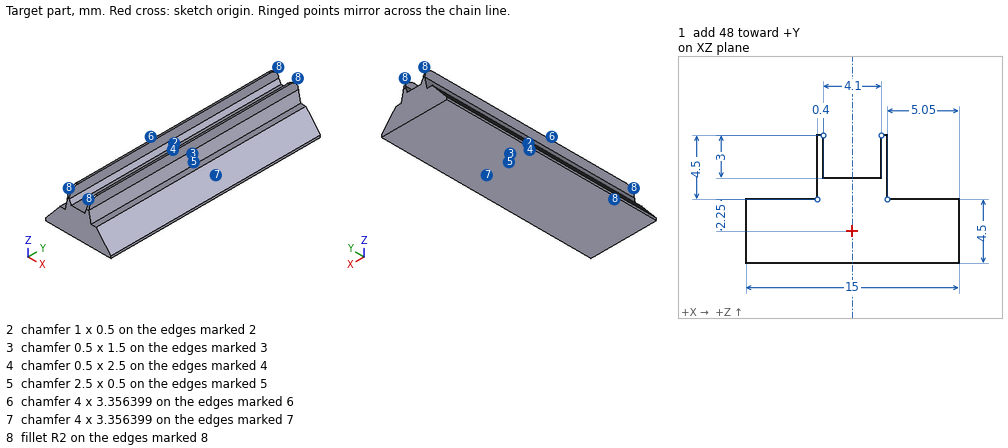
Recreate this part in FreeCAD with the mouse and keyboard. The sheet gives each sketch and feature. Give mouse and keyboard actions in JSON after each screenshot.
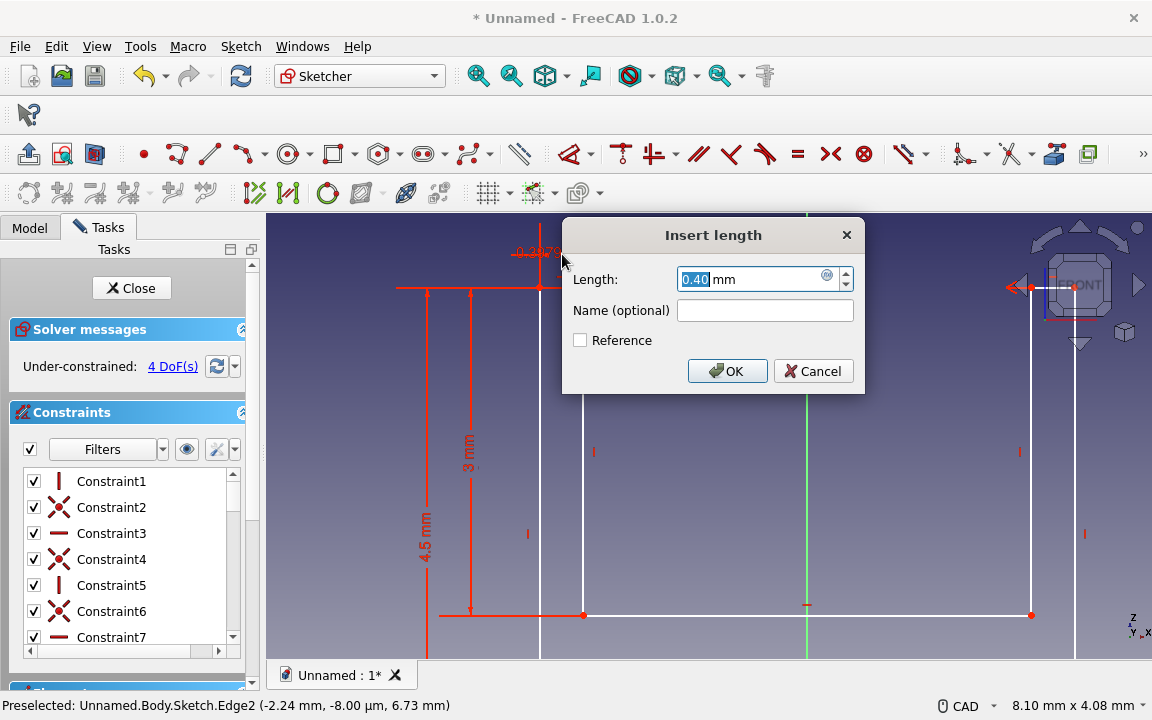
{"action": "type", "text": "0.4"}
{"action": "key", "text": "Return"}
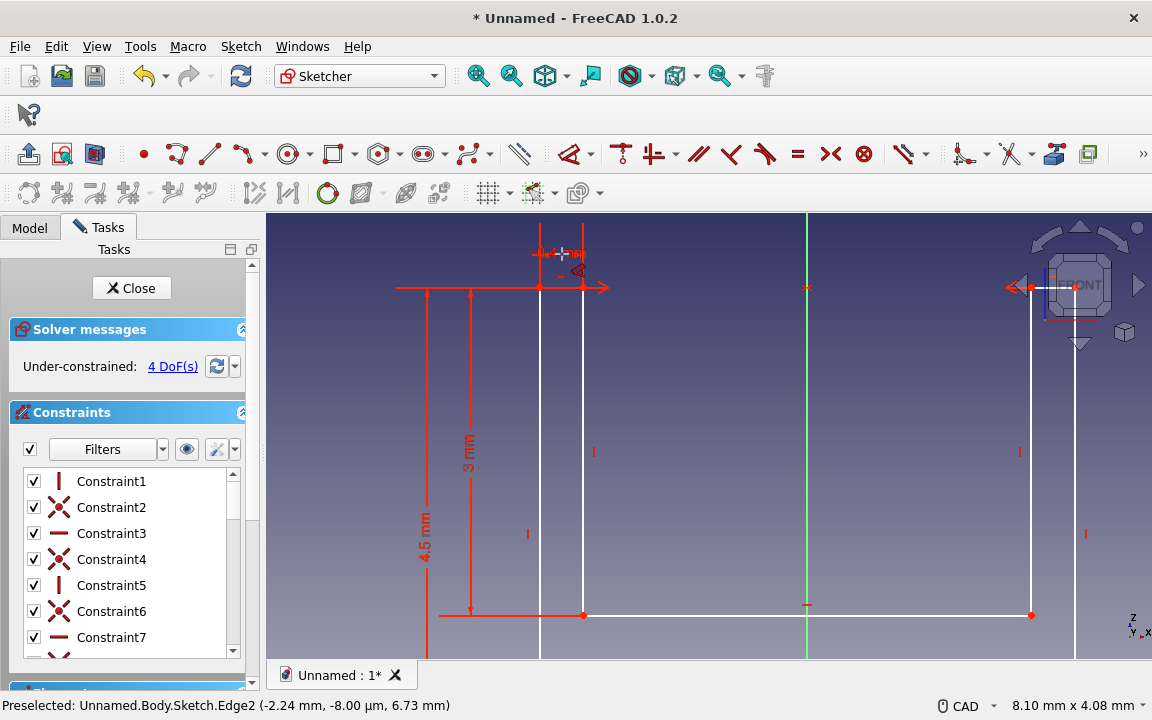
{"action": "left_click", "coordinate": [718, 616]}
{"action": "left_click", "coordinate": [785, 582]}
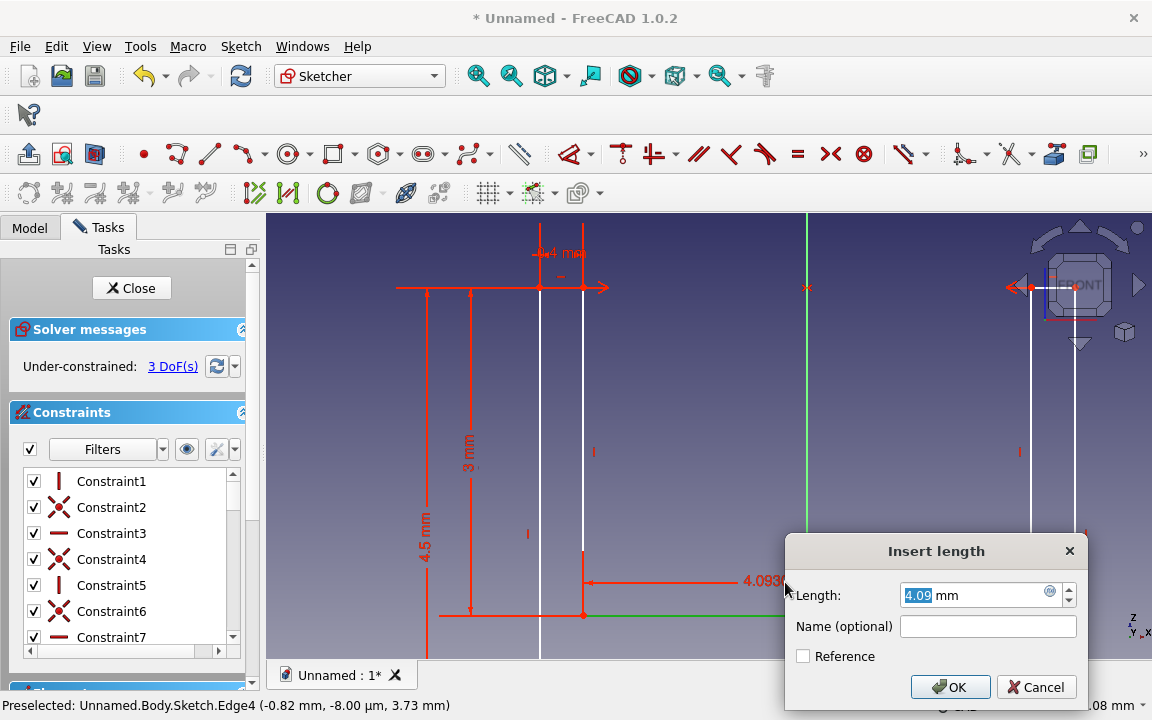
{"action": "type", "text": "4.1"}
{"action": "key", "text": "Return"}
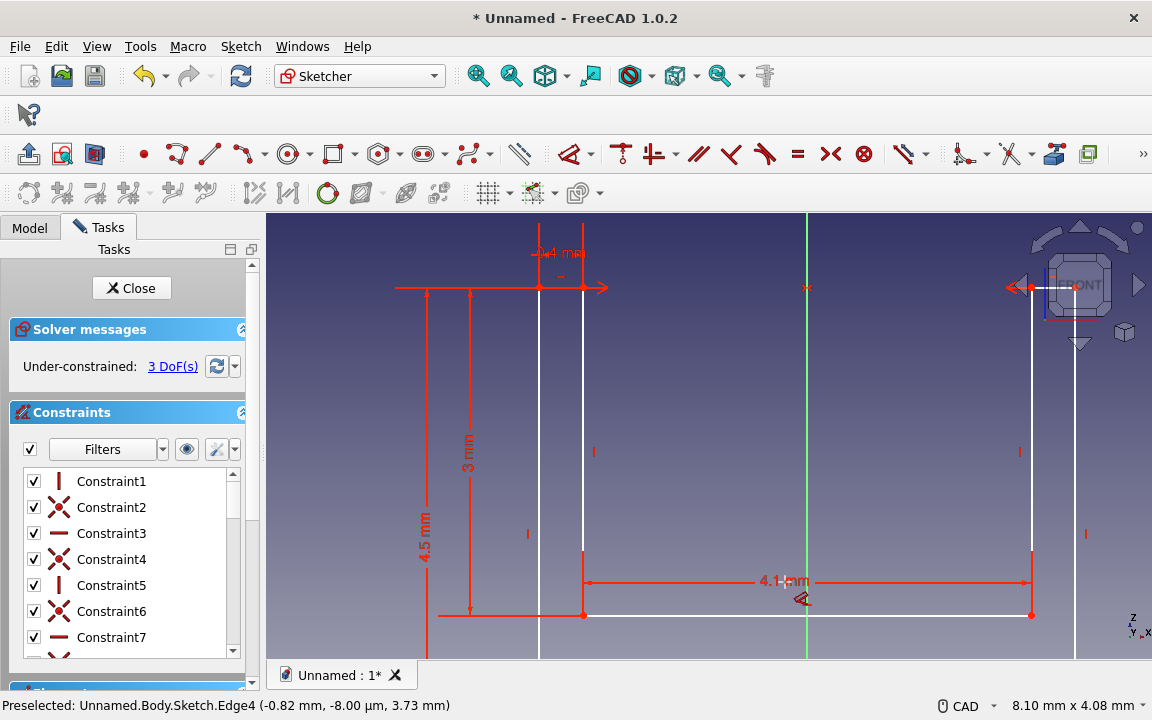
{"action": "scroll", "coordinate": [569, 289], "scroll_direction": "down", "scroll_amount": 6}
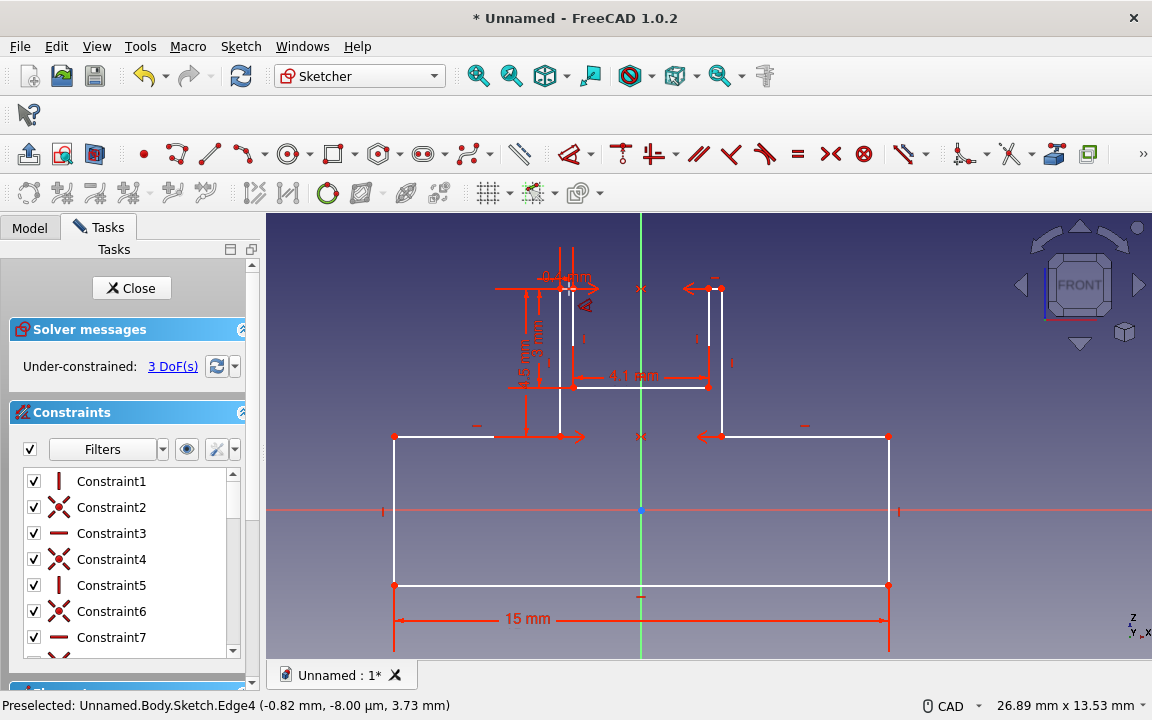
{"action": "left_click", "coordinate": [889, 482]}
{"action": "left_click", "coordinate": [923, 477]}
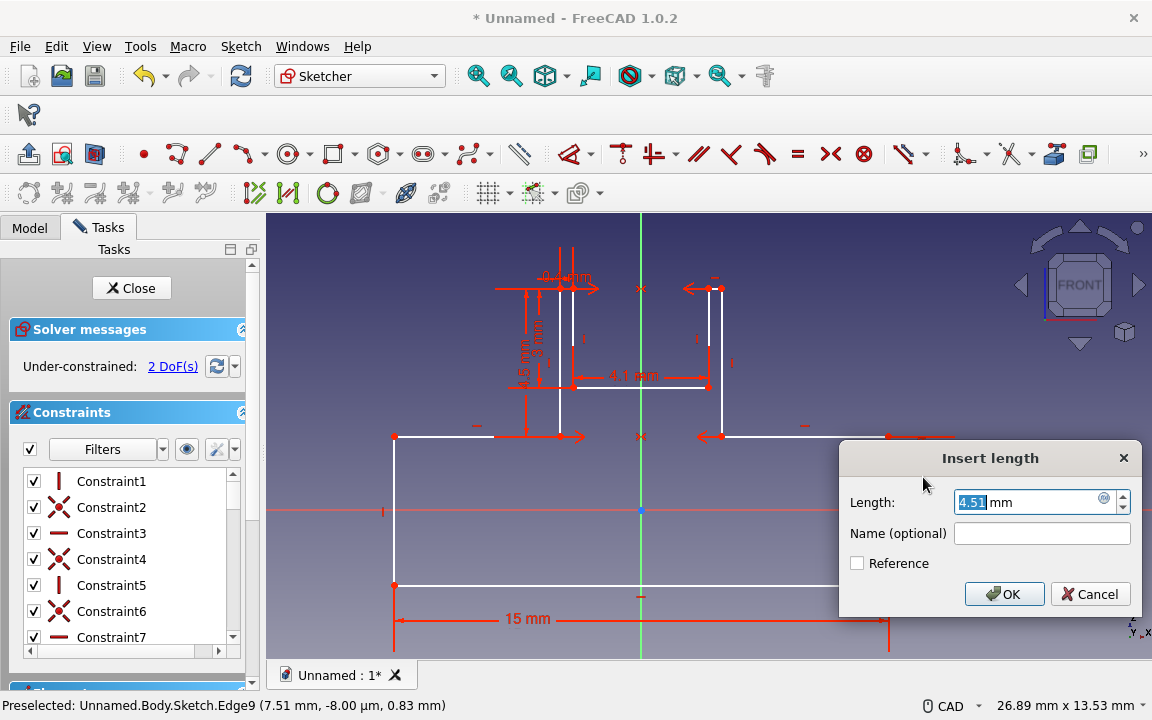
{"action": "type", "text": "4.5"}
{"action": "key", "text": "Return"}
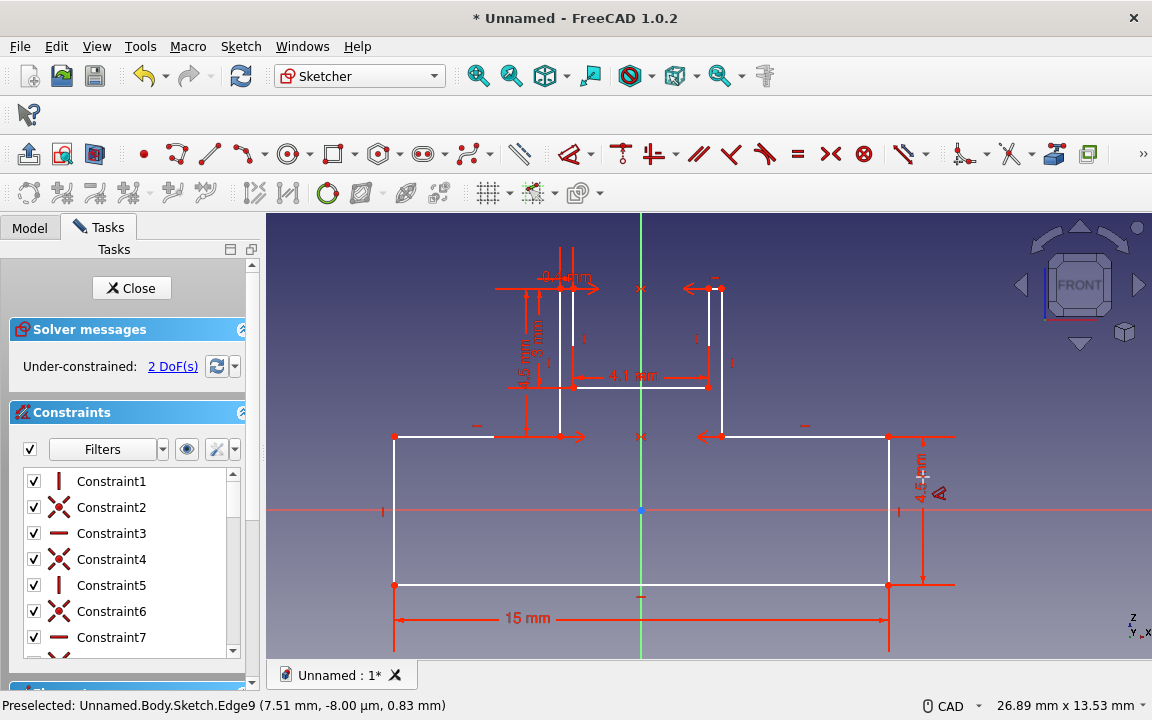
{"action": "left_click", "coordinate": [772, 437]}
{"action": "left_click", "coordinate": [805, 471]}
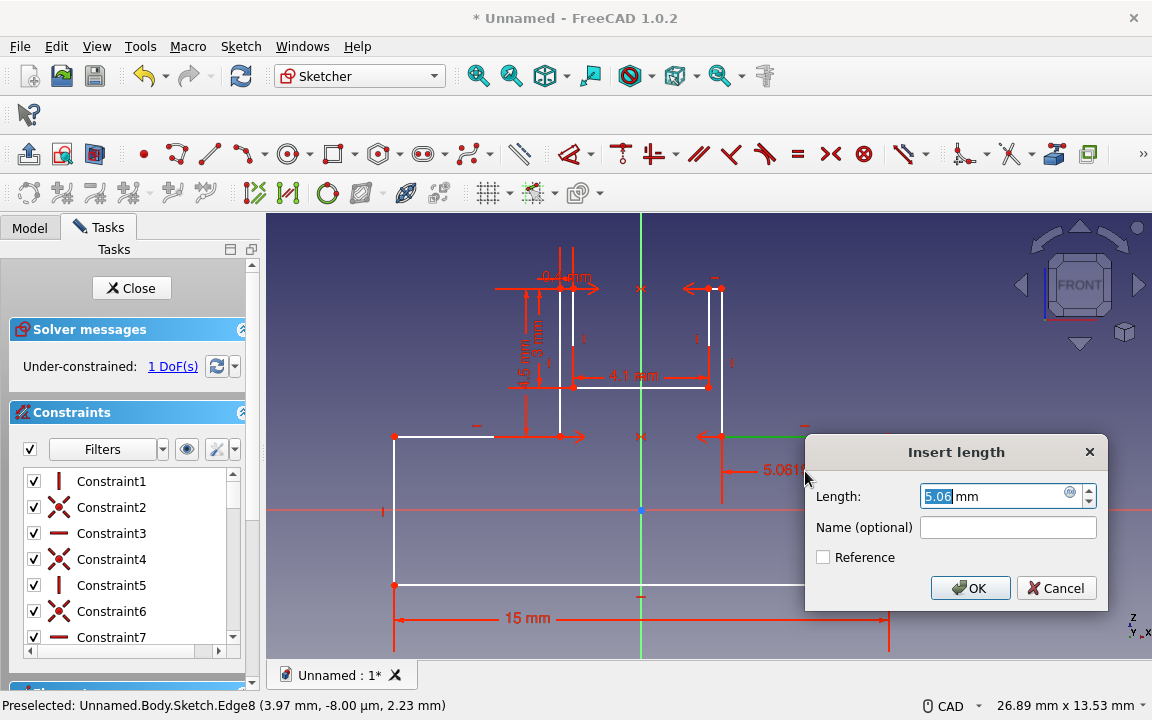
{"action": "type", "text": "5.05"}
{"action": "key", "text": "Return"}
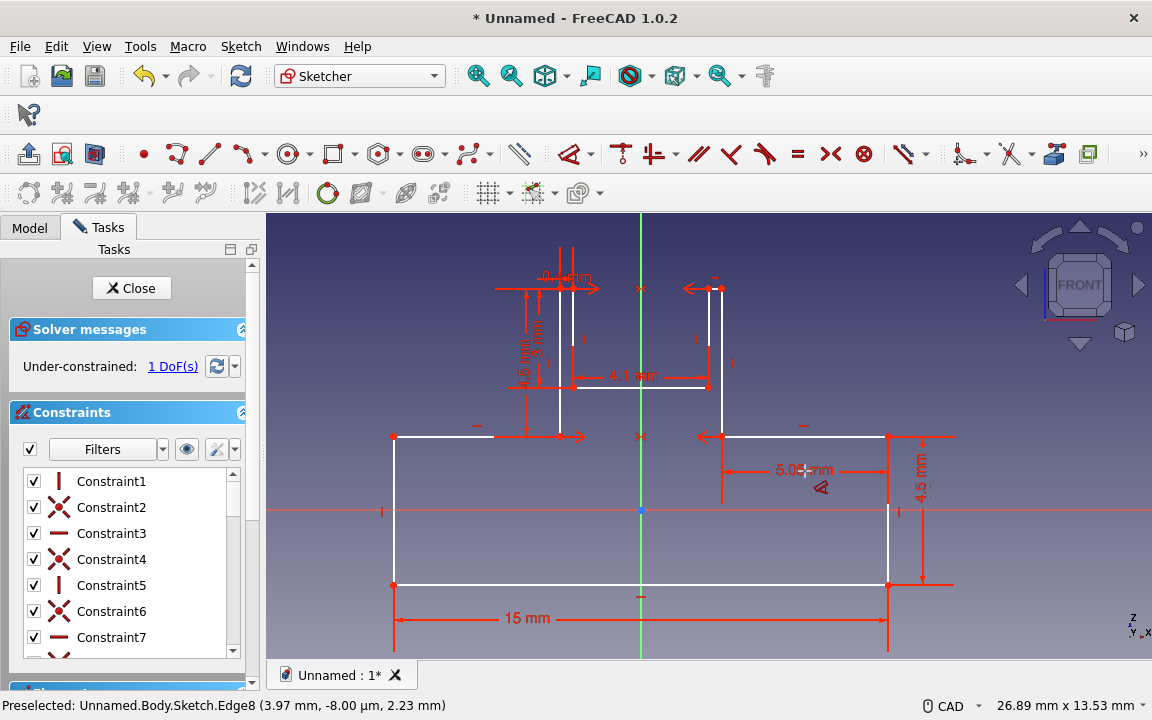
{"action": "left_click", "coordinate": [560, 437]}
{"action": "left_click", "coordinate": [526, 474]}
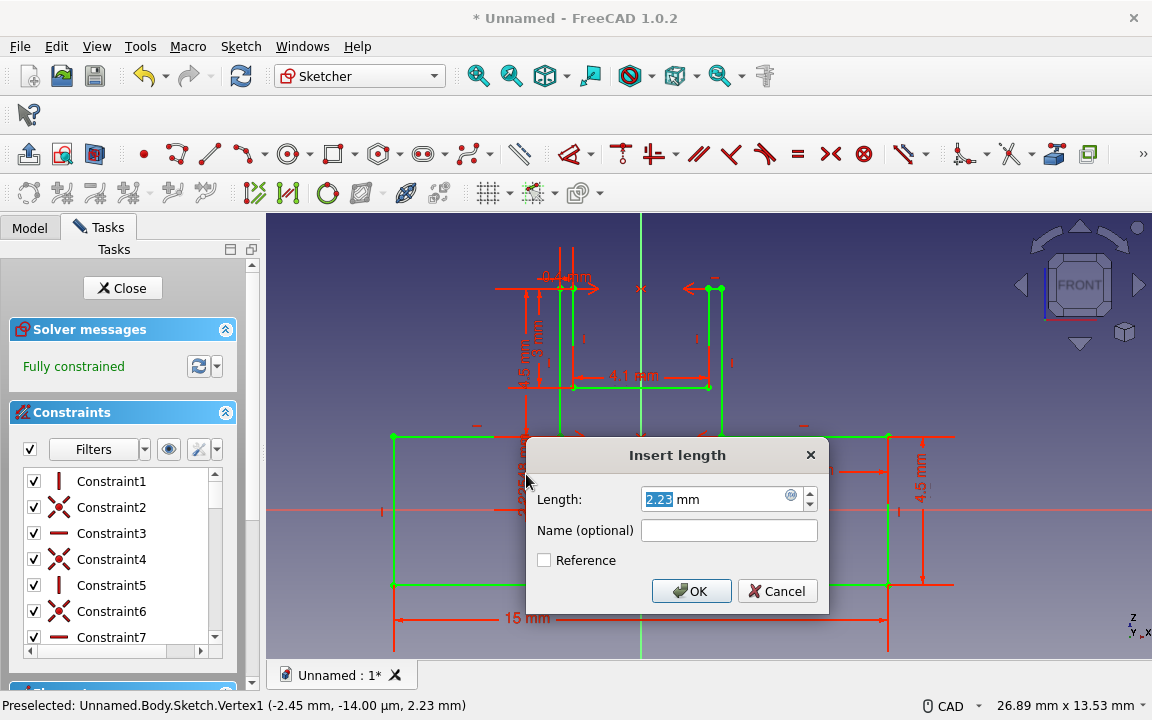
{"action": "type", "text": "2.25"}
{"action": "key", "text": "Return"}
{"action": "key", "text": "Escape"}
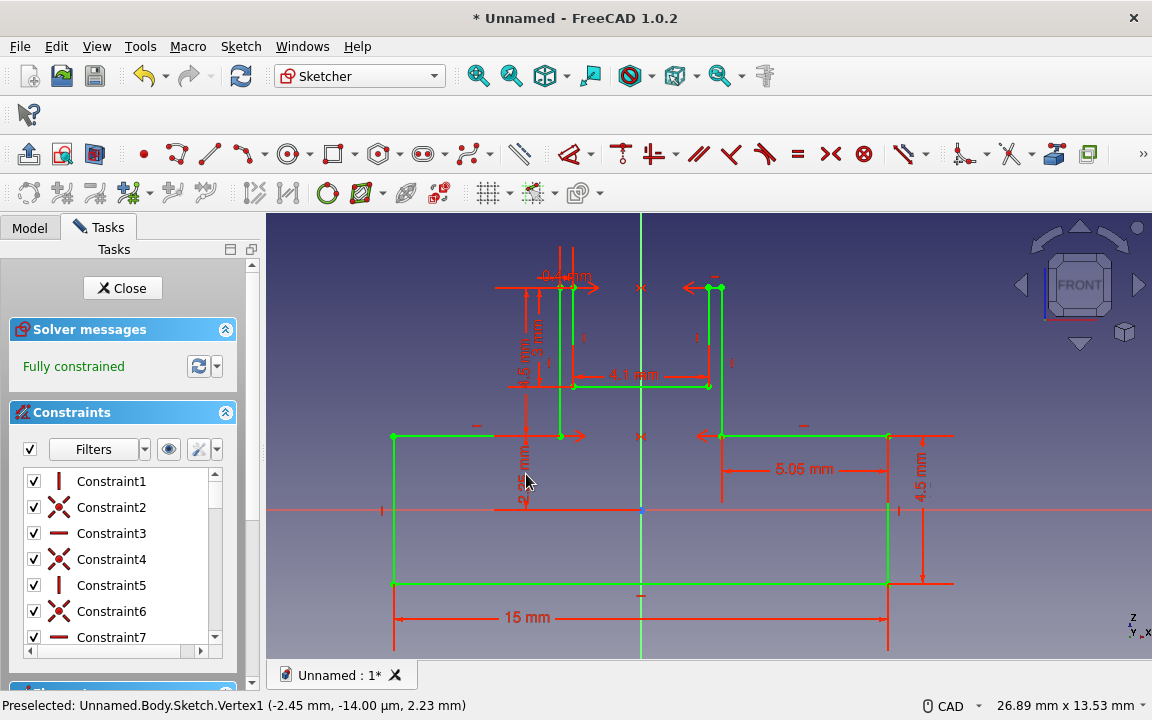
{"action": "left_click", "coordinate": [123, 288]}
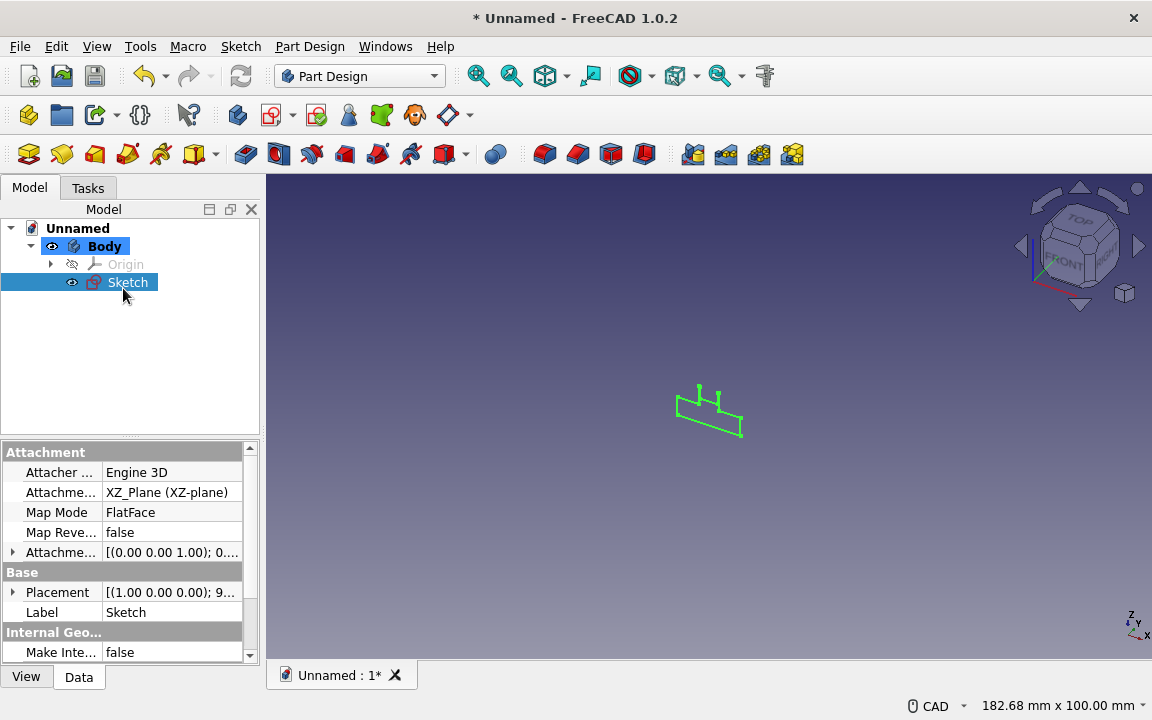
{"action": "left_click", "coordinate": [29, 154]}